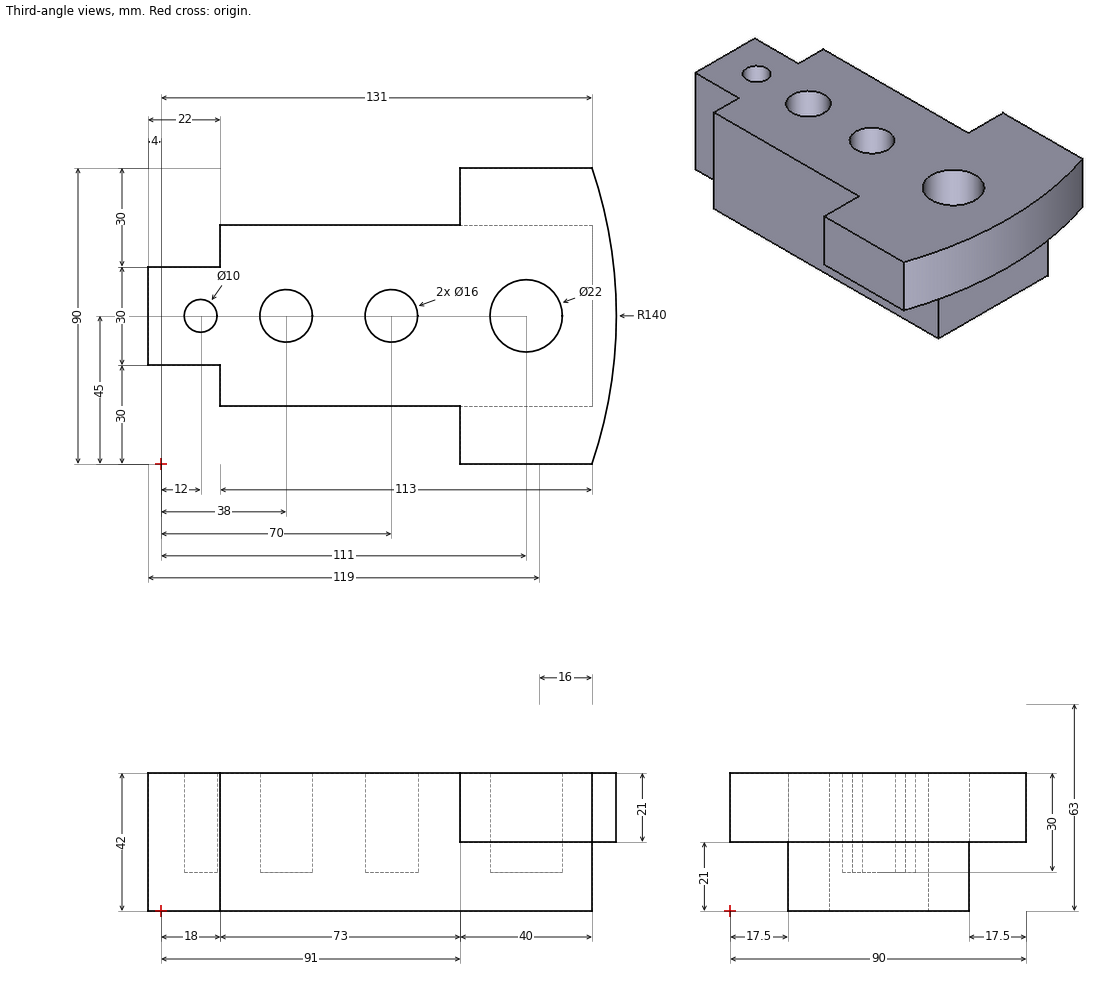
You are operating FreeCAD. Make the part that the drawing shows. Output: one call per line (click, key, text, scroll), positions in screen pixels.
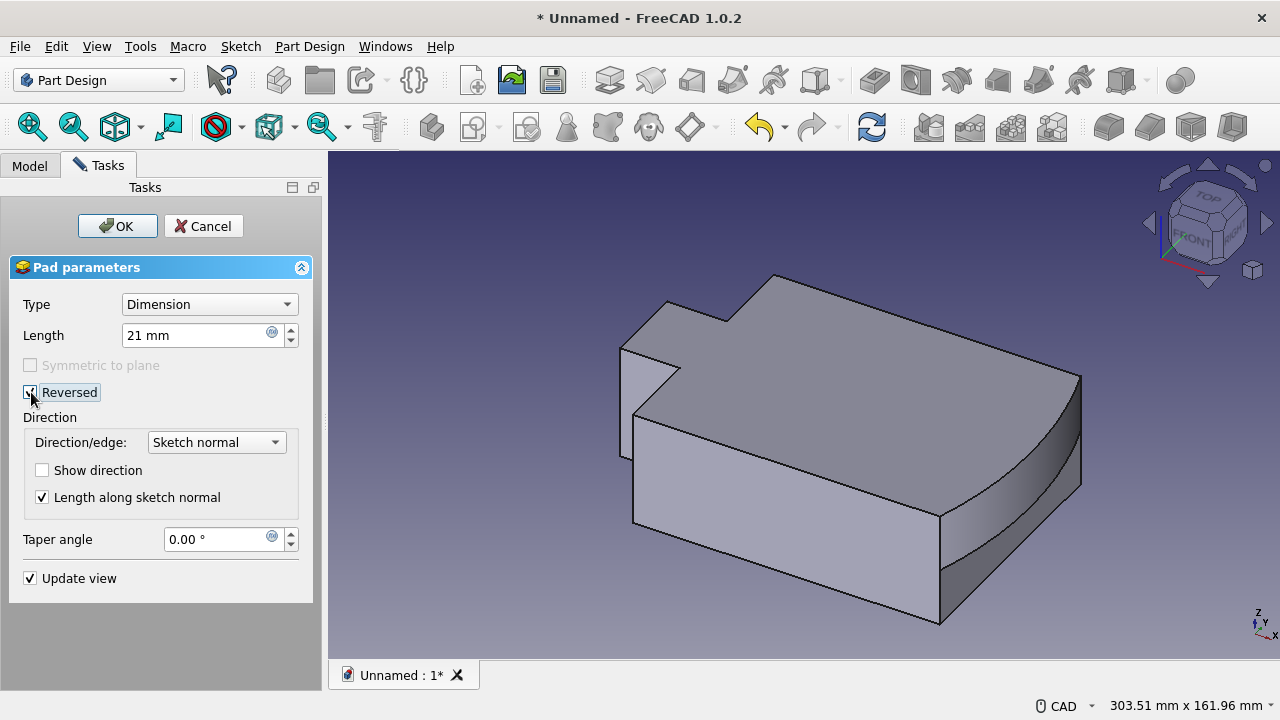
click(118, 226)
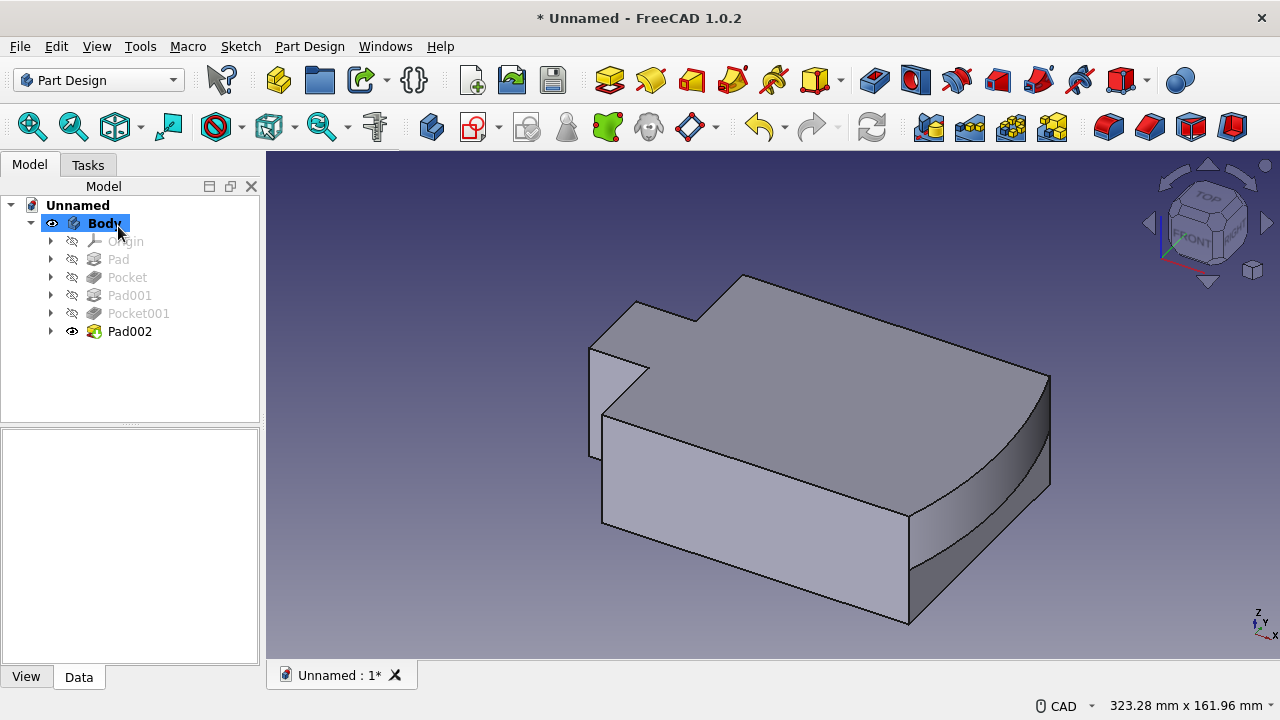
click(939, 566)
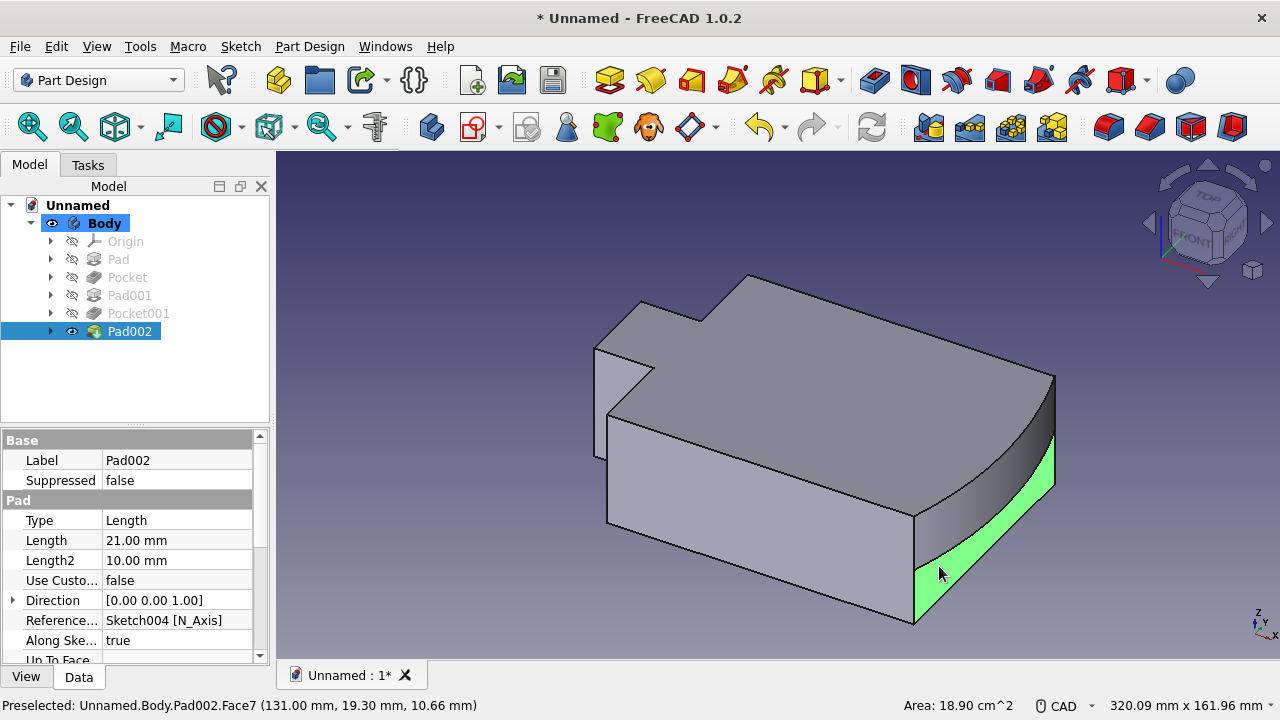
click(472, 128)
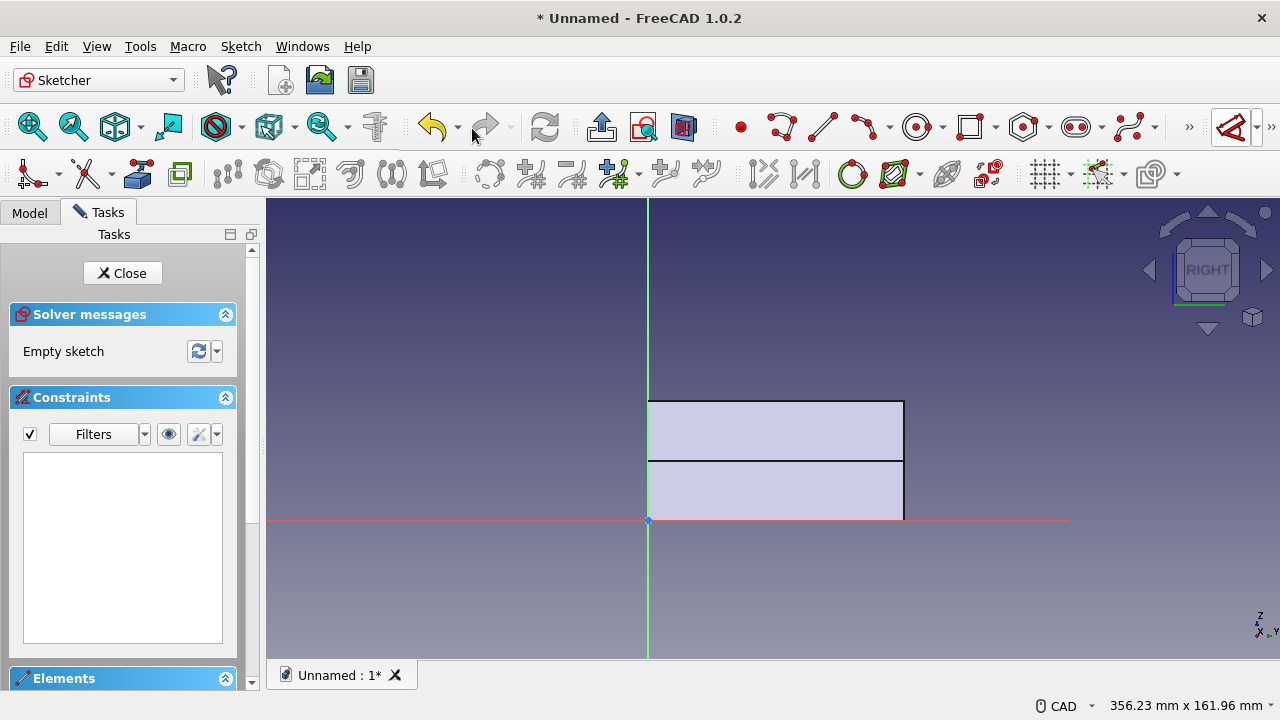
scroll(835, 542, up, 4)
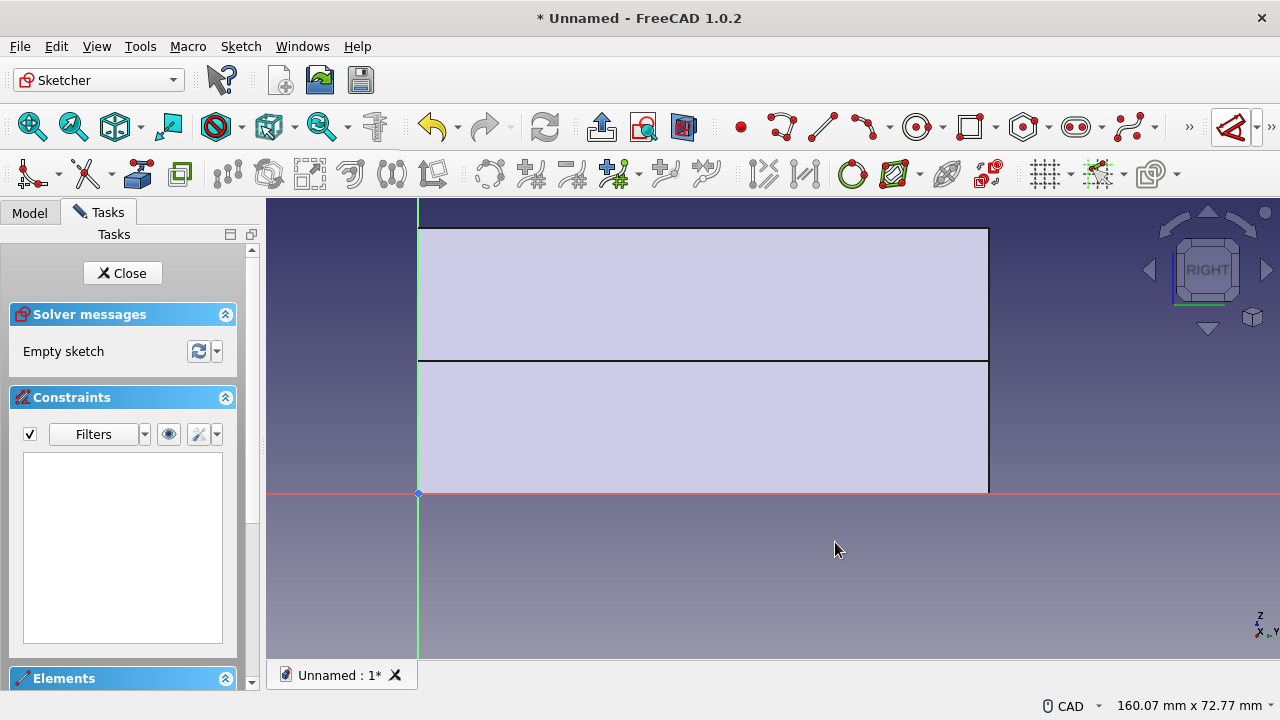
click(970, 128)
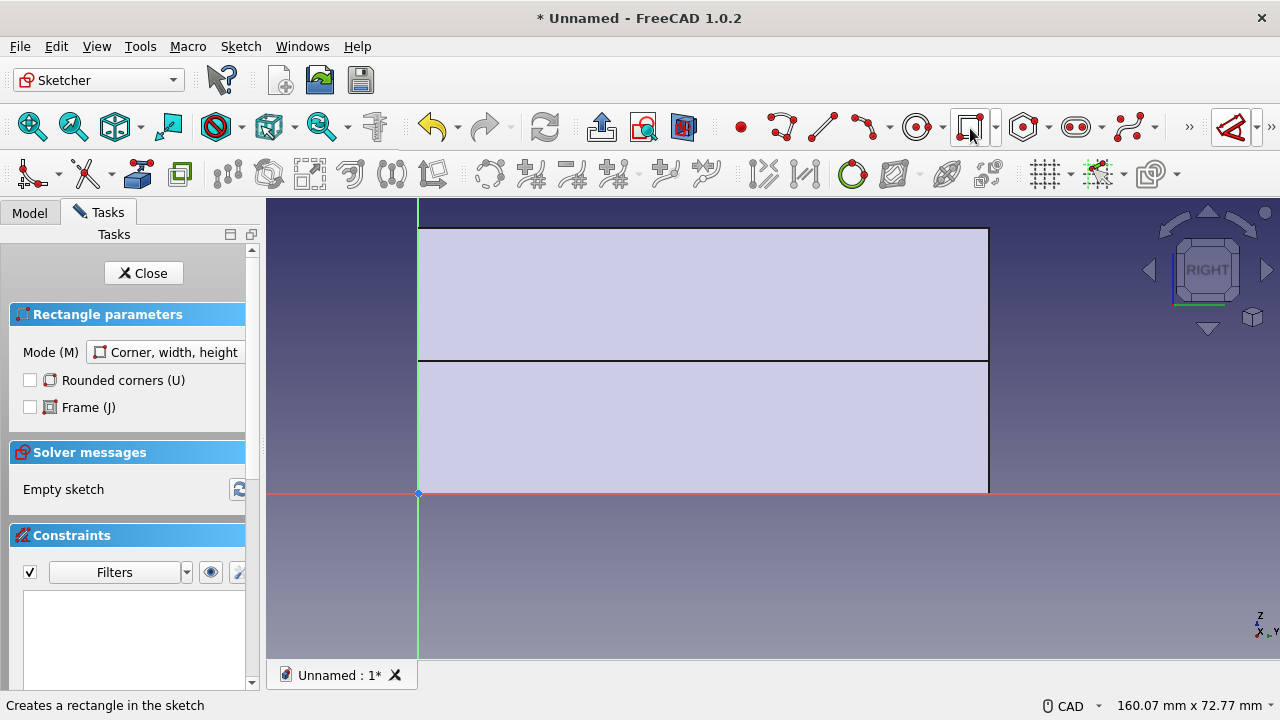
click(878, 361)
click(989, 494)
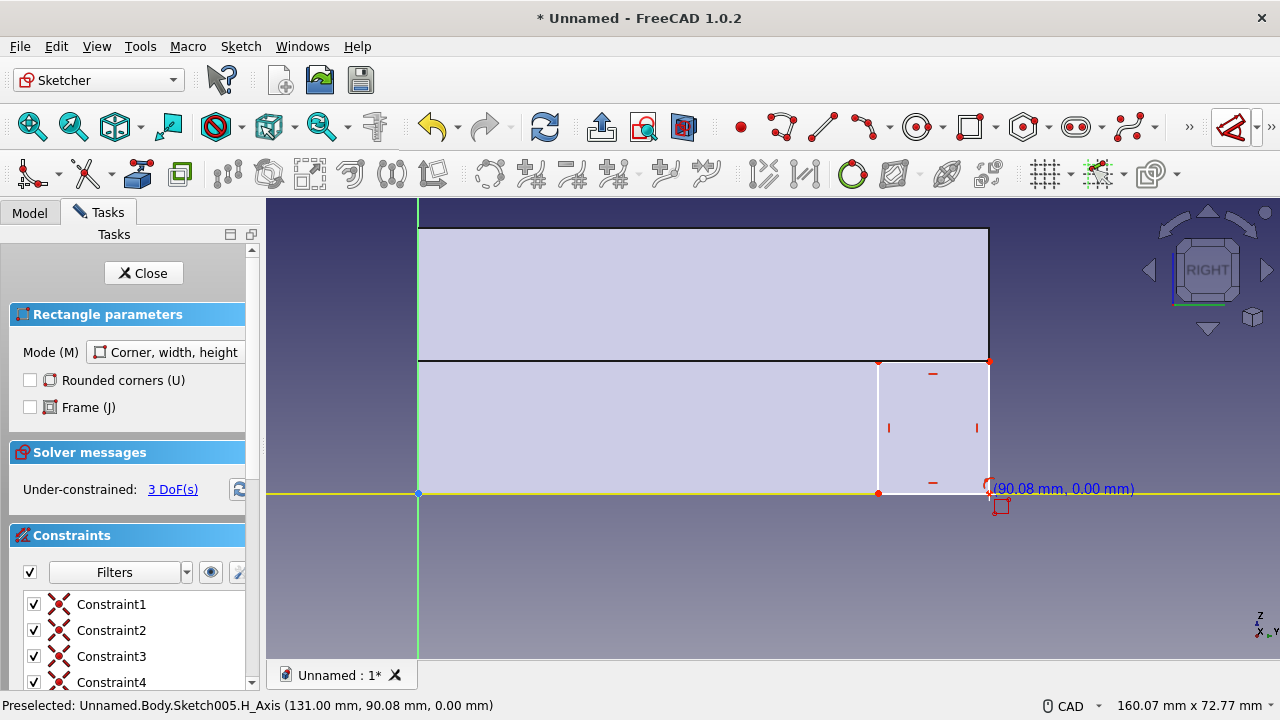
click(418, 494)
move(529, 361)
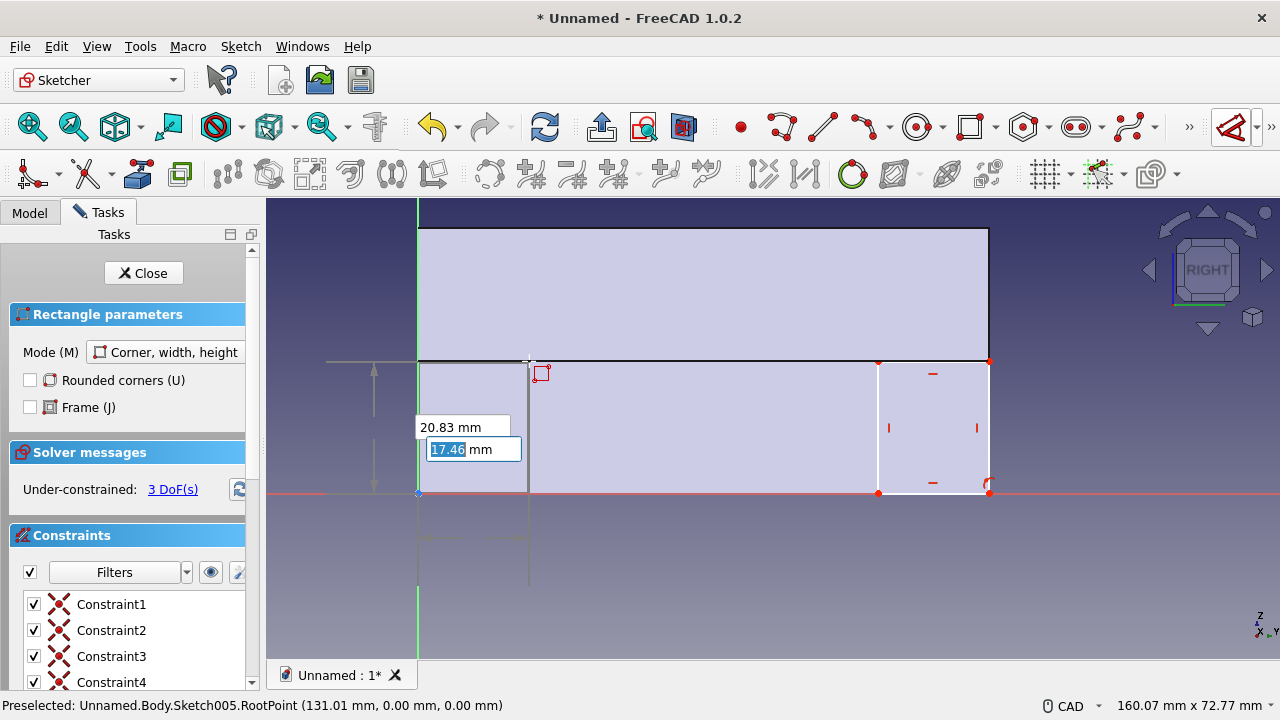
text(17.5)
key(Tab)
text(21)
key(Return)
key(Escape)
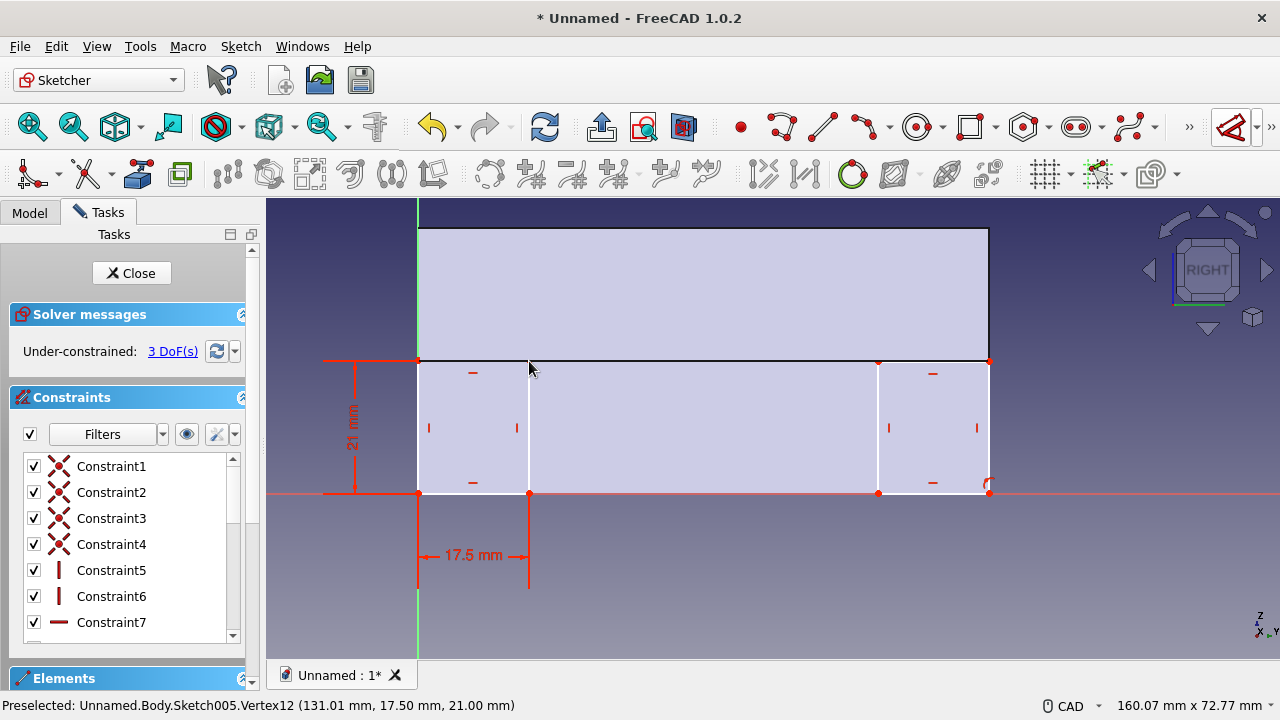
click(878, 402)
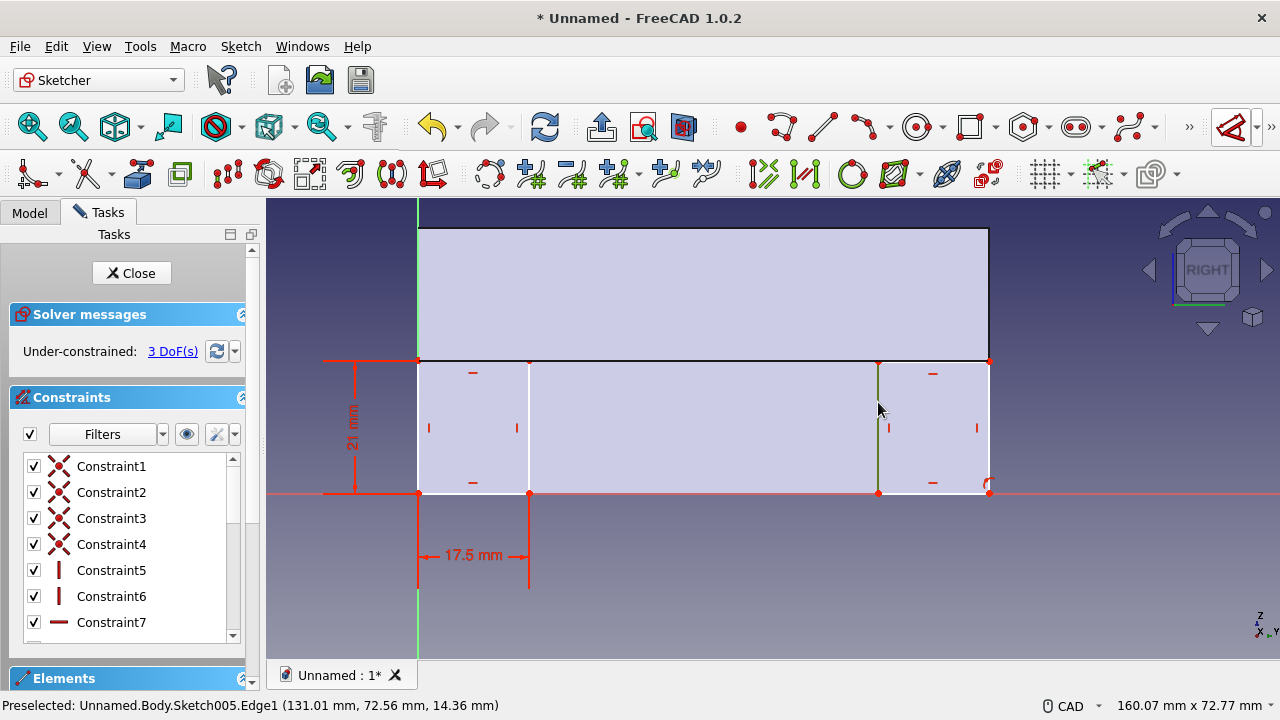
click(1256, 128)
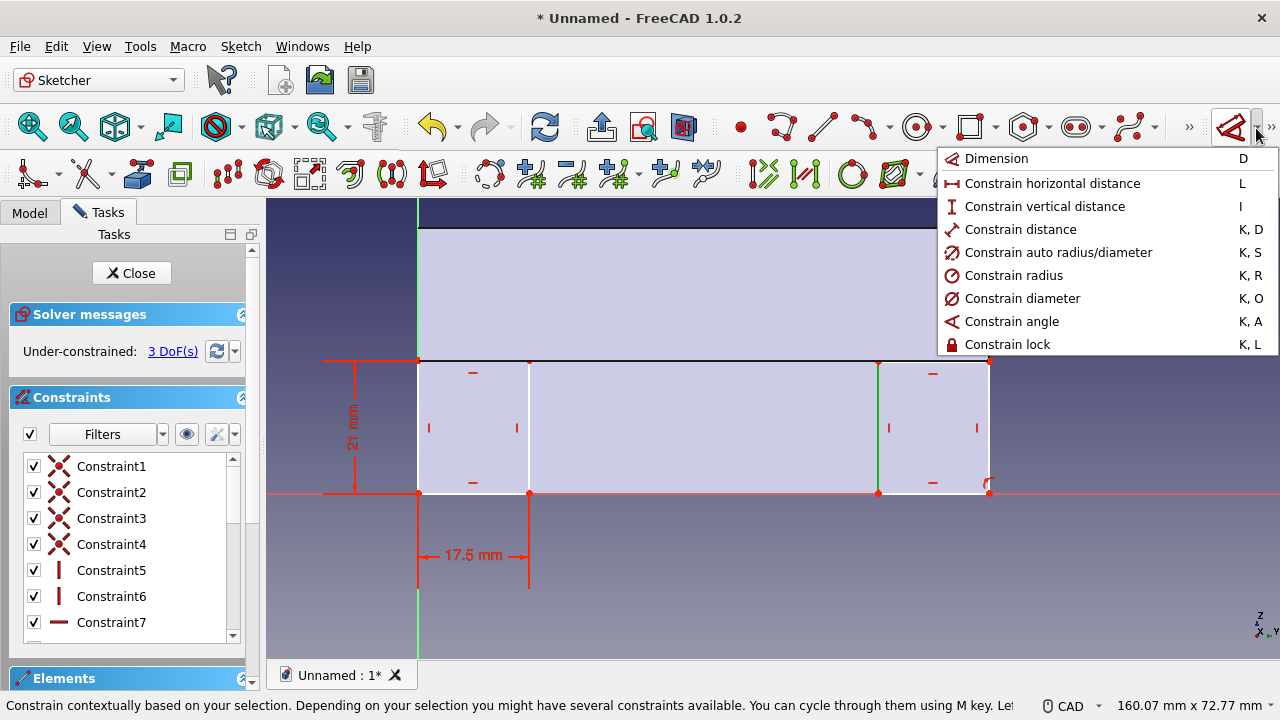
click(1108, 206)